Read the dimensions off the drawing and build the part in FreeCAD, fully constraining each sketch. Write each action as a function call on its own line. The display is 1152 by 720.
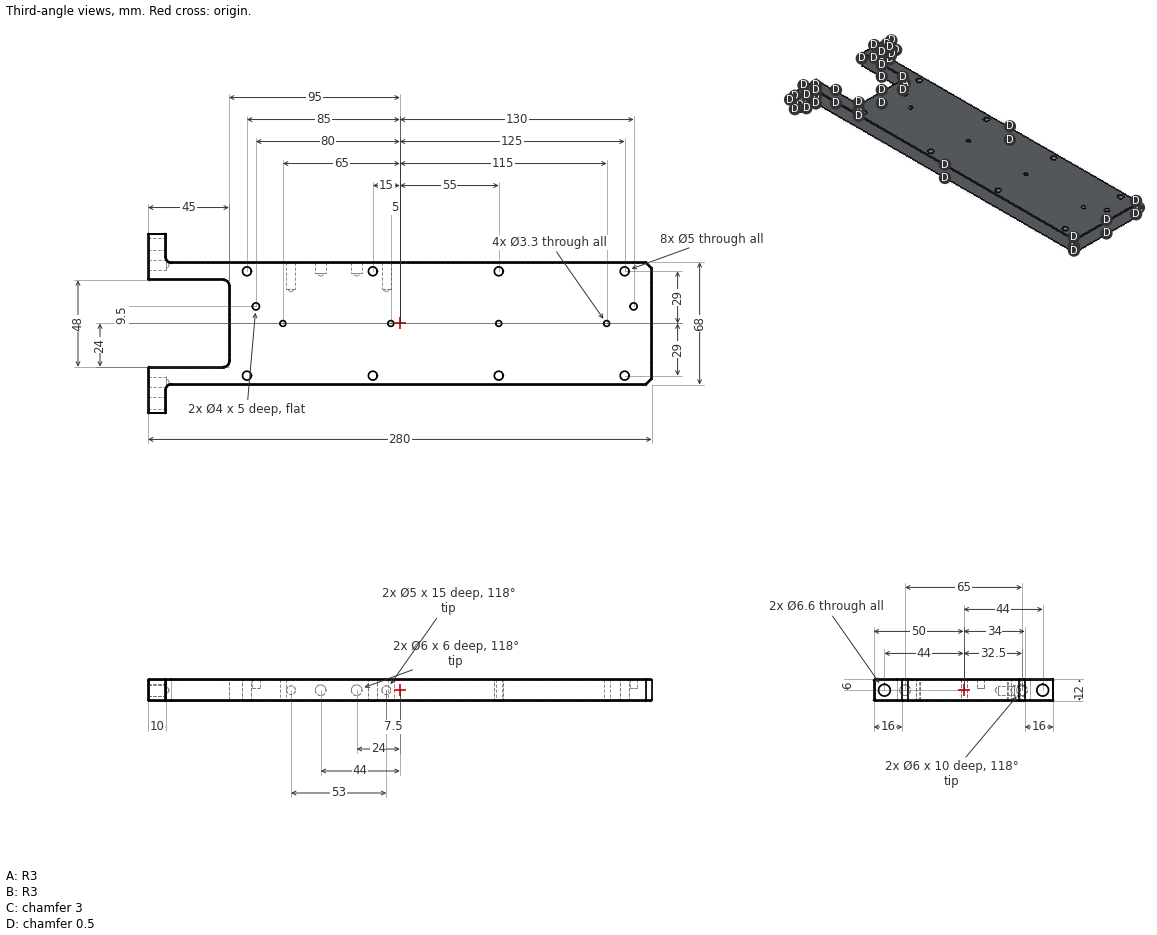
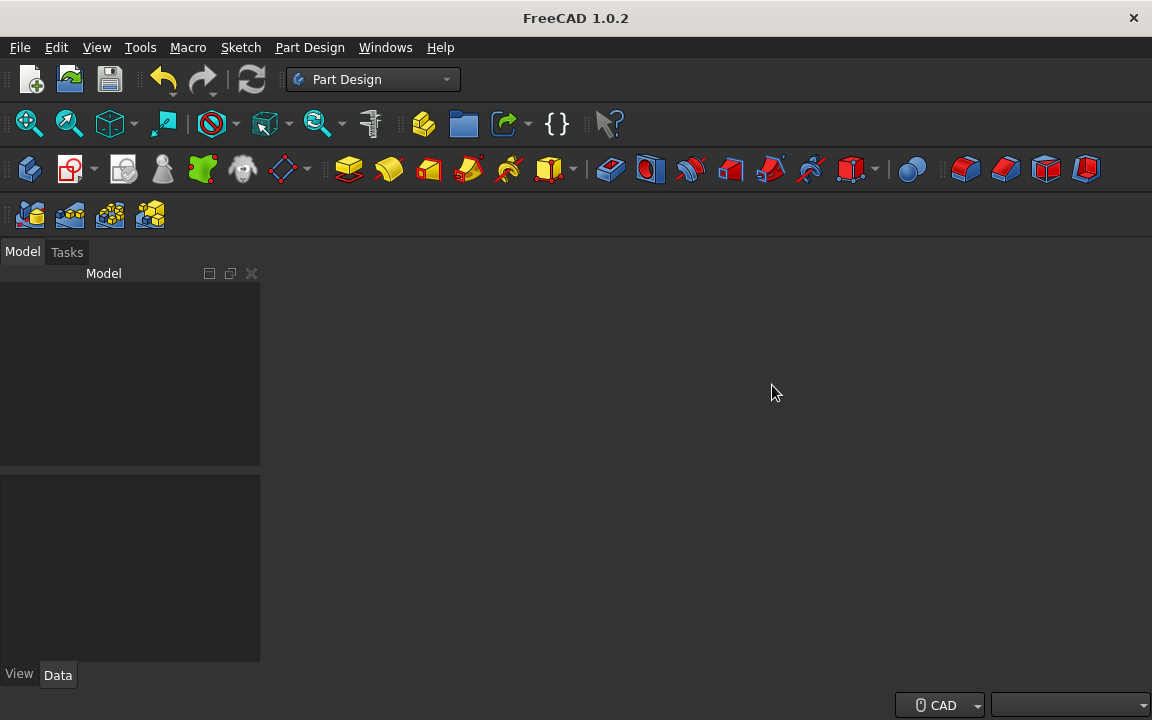
key(ctrl+n)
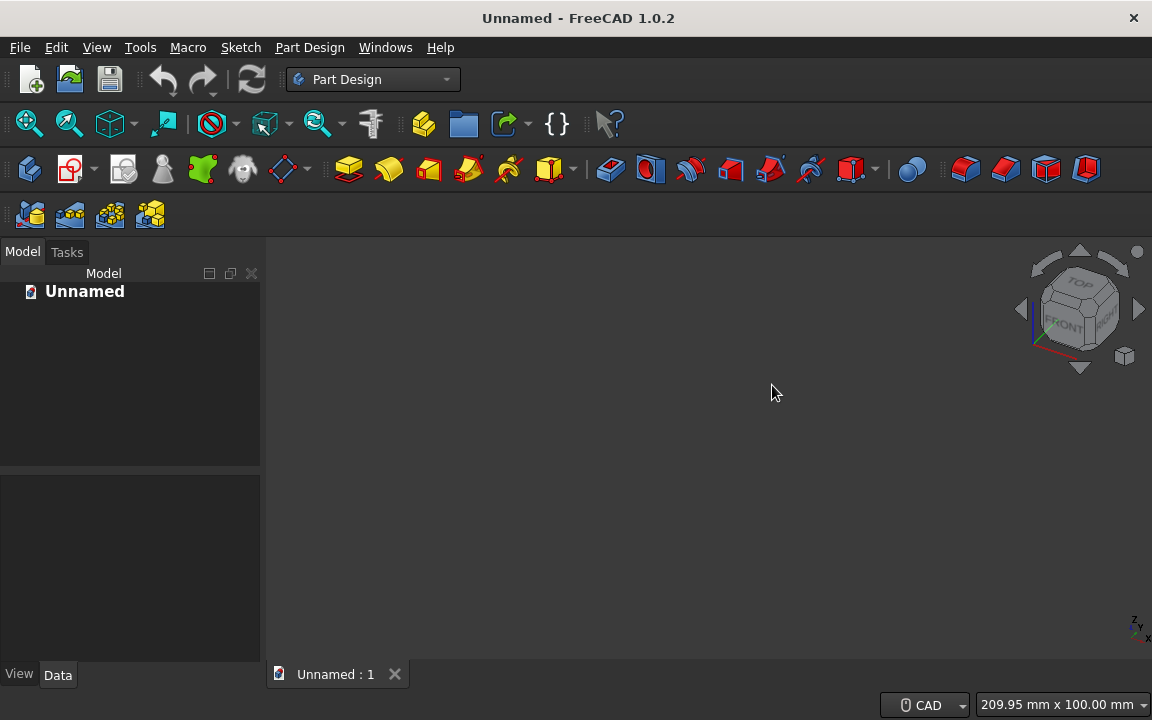
click(70, 170)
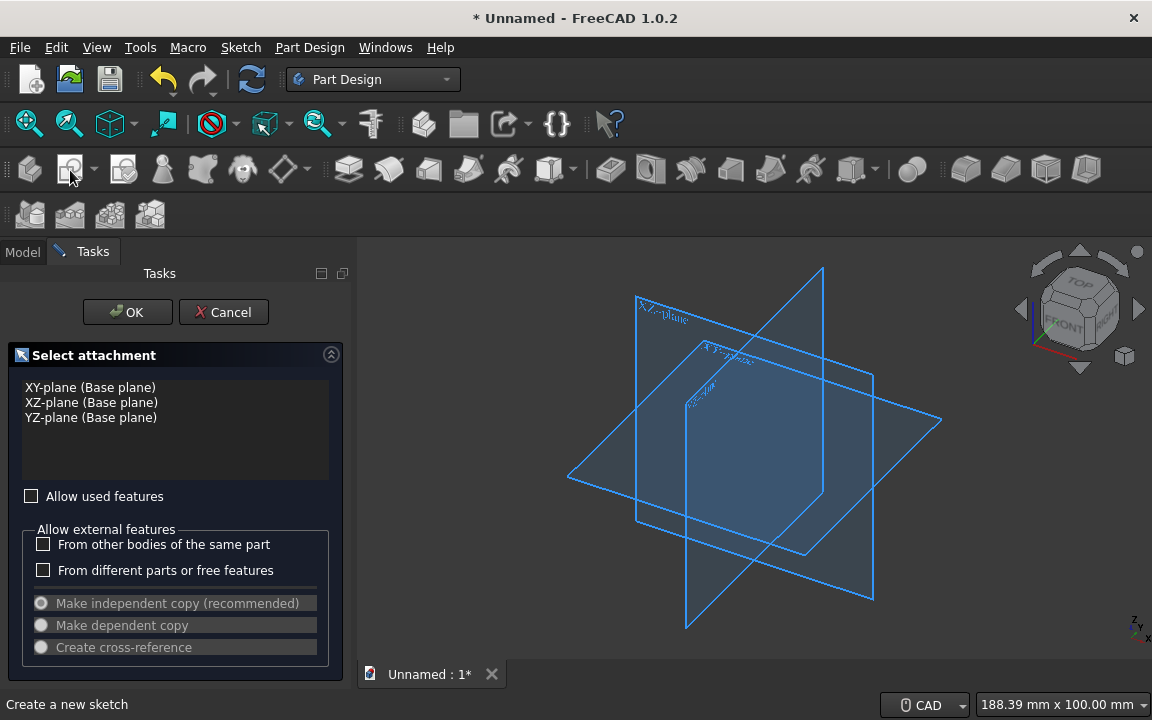
click(82, 388)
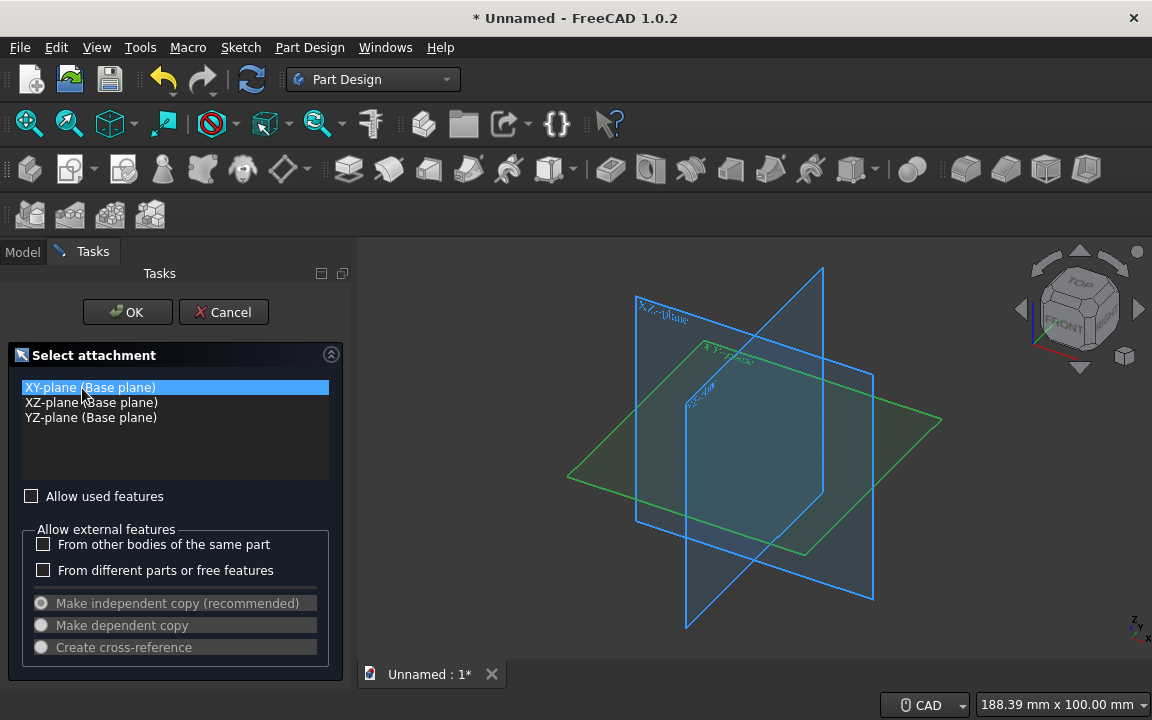
click(128, 312)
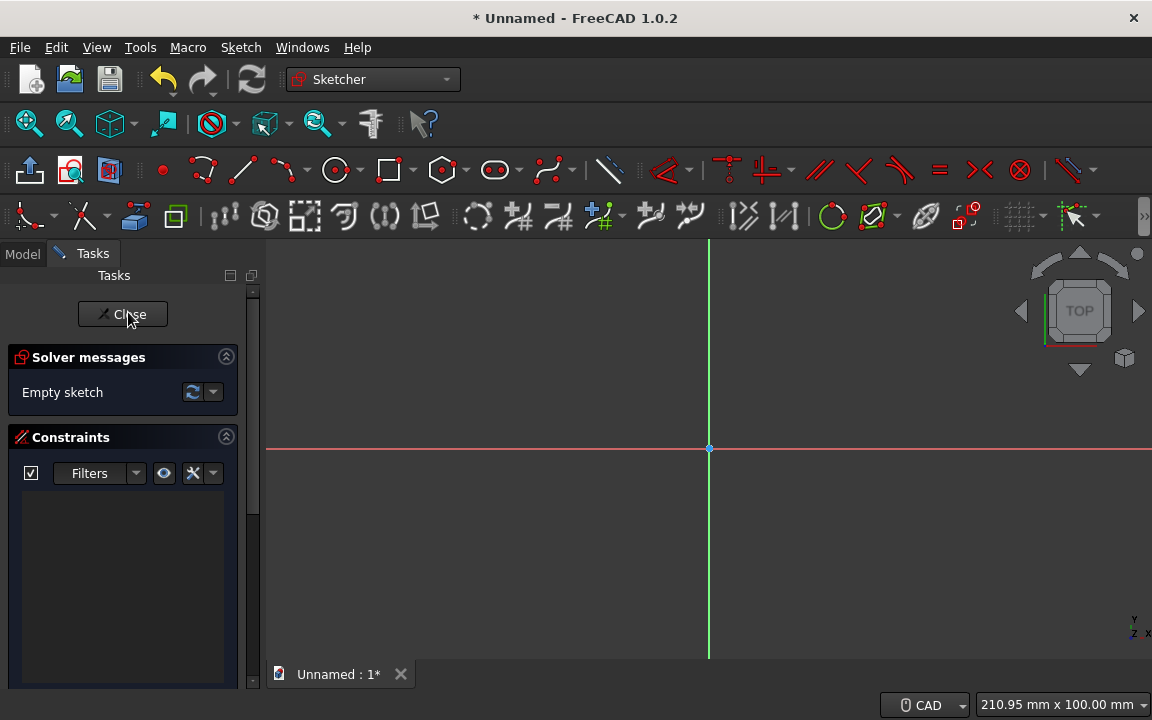
scroll(585, 449, down, 4)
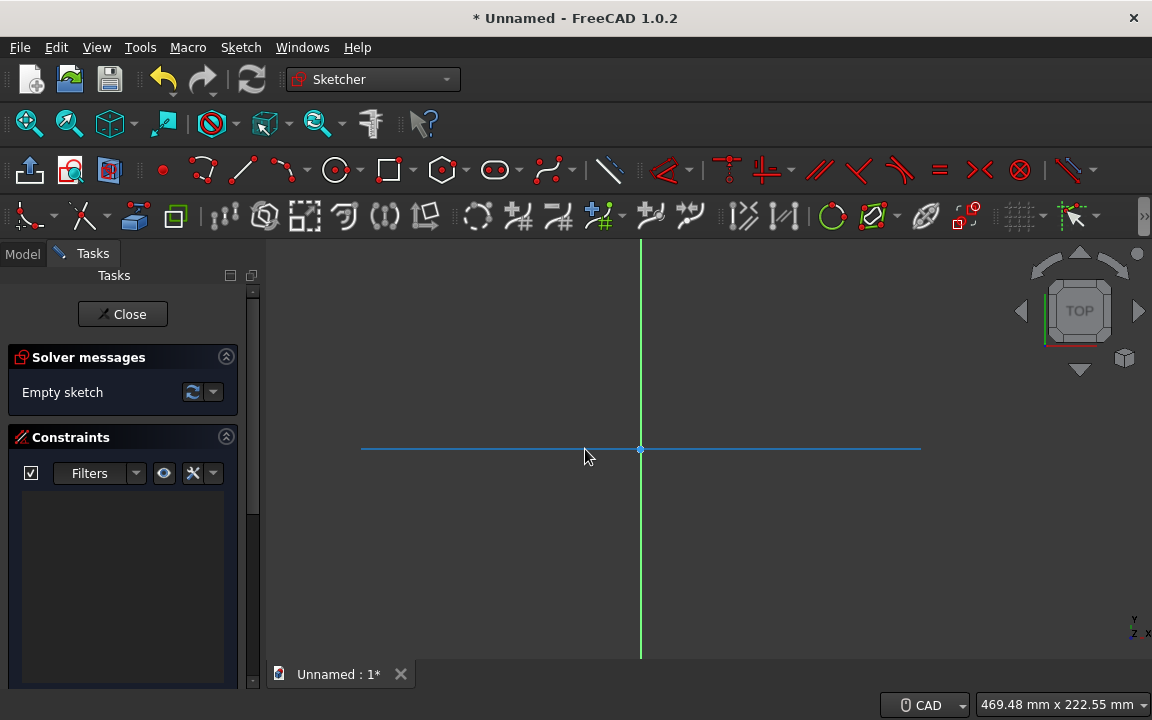
key(g)
key(v)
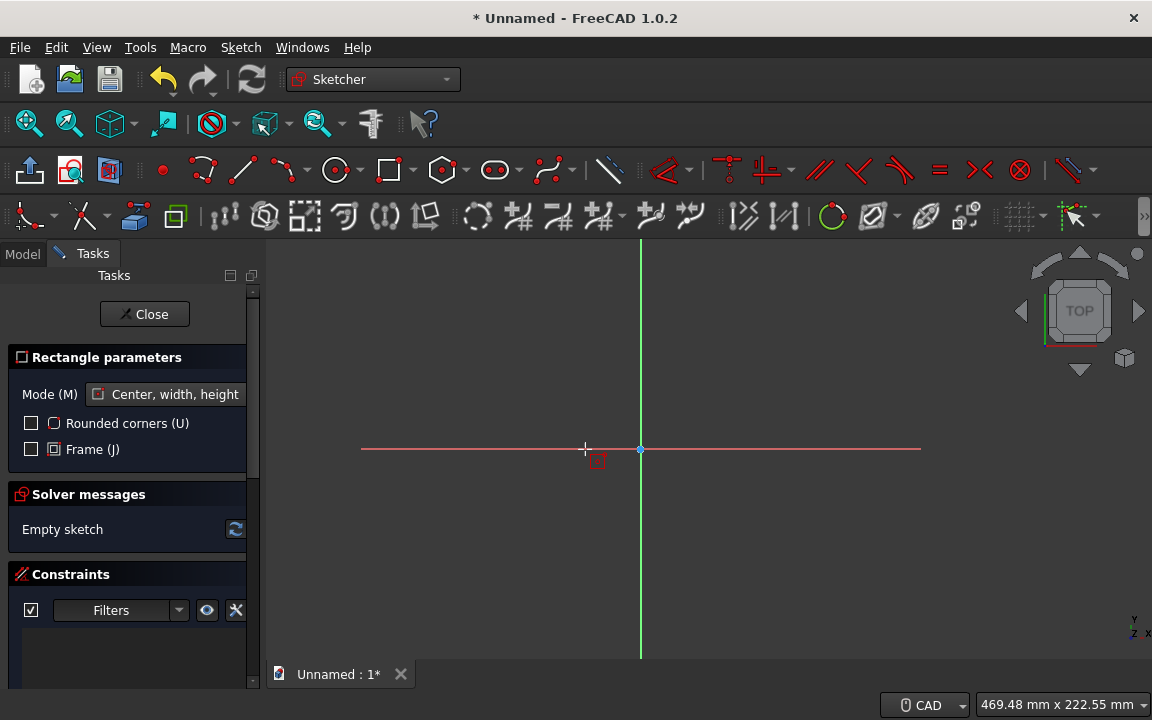
click(641, 449)
move(905, 385)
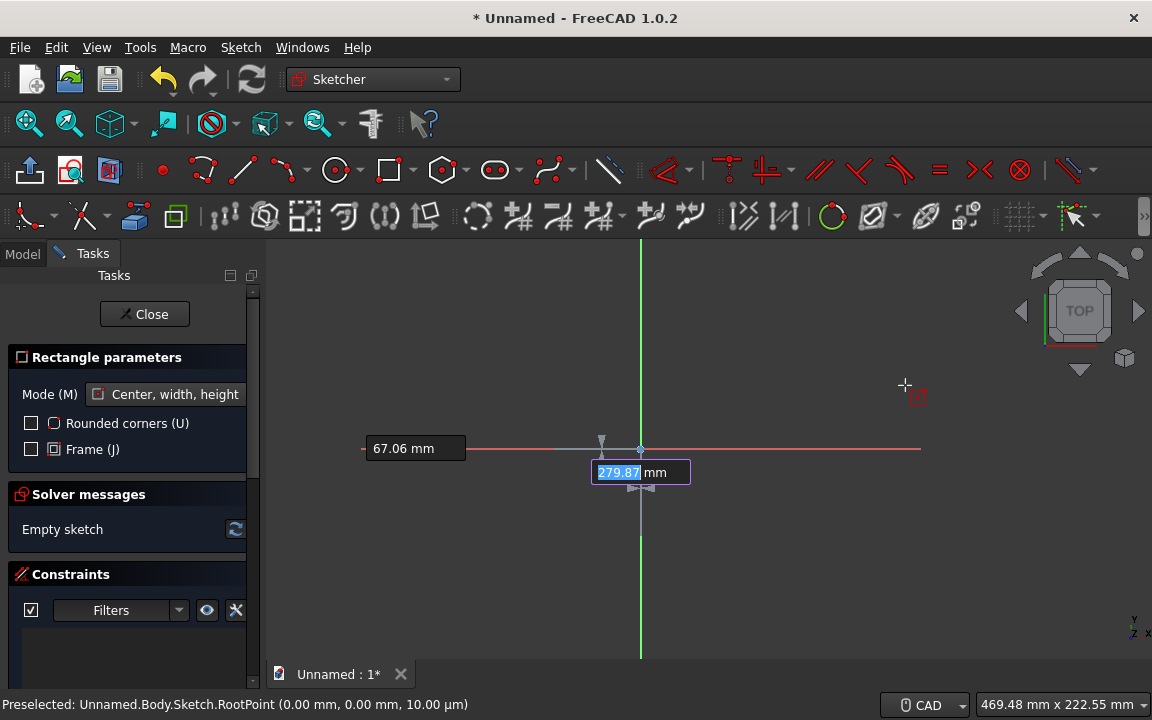
text(280)
key(Tab)
text(68)
key(Return)
key(Escape)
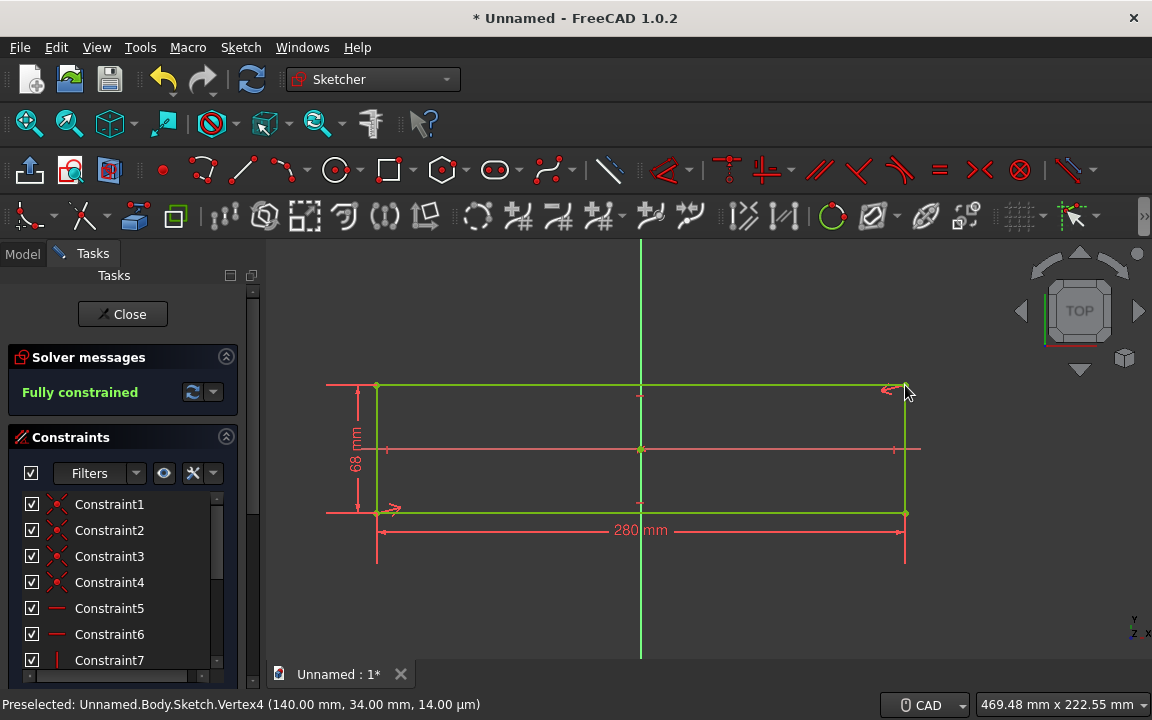
click(123, 314)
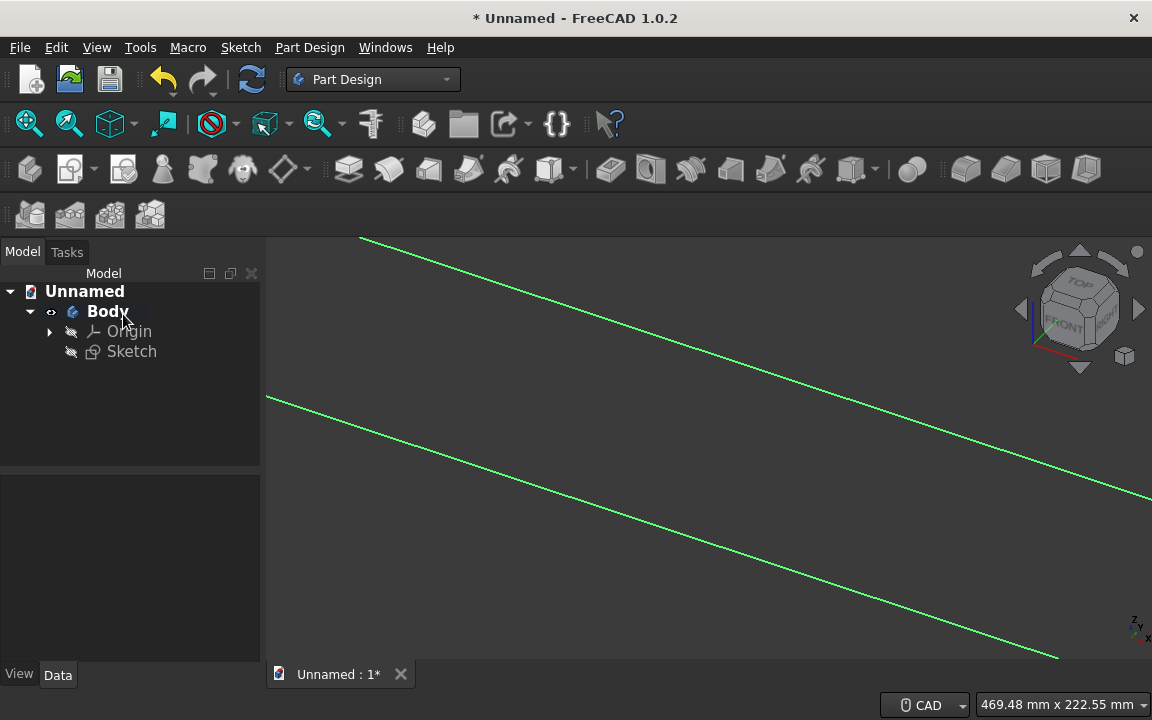
click(350, 170)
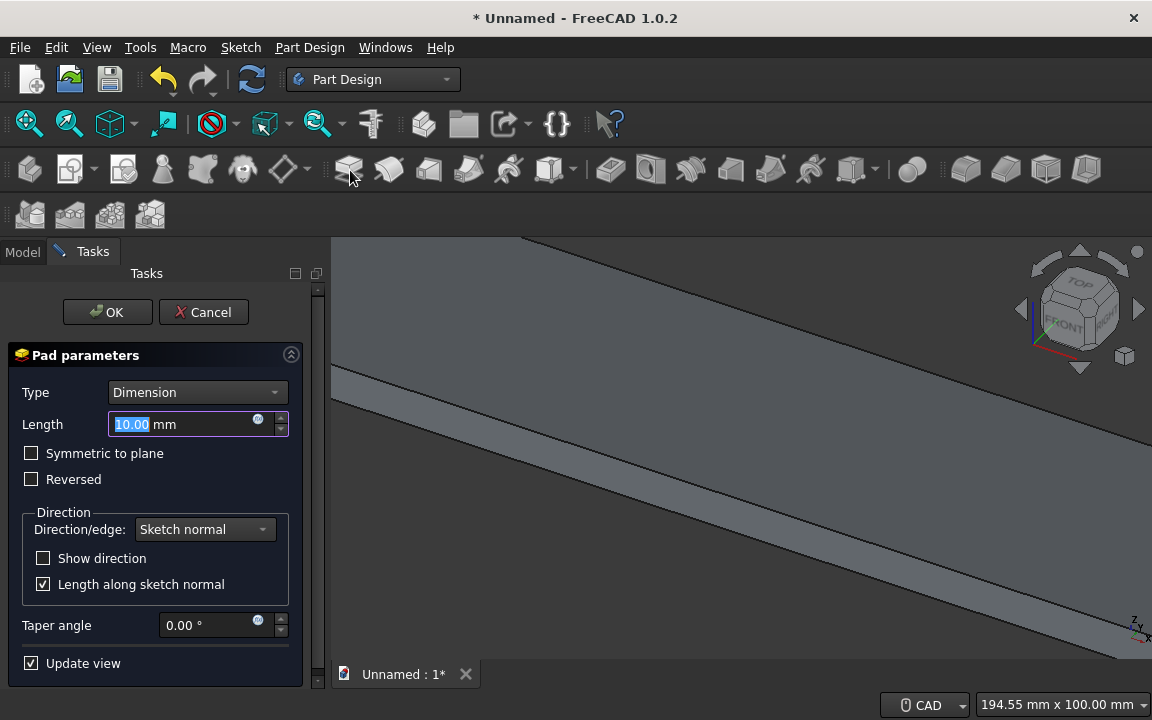
text(12)
key(Tab)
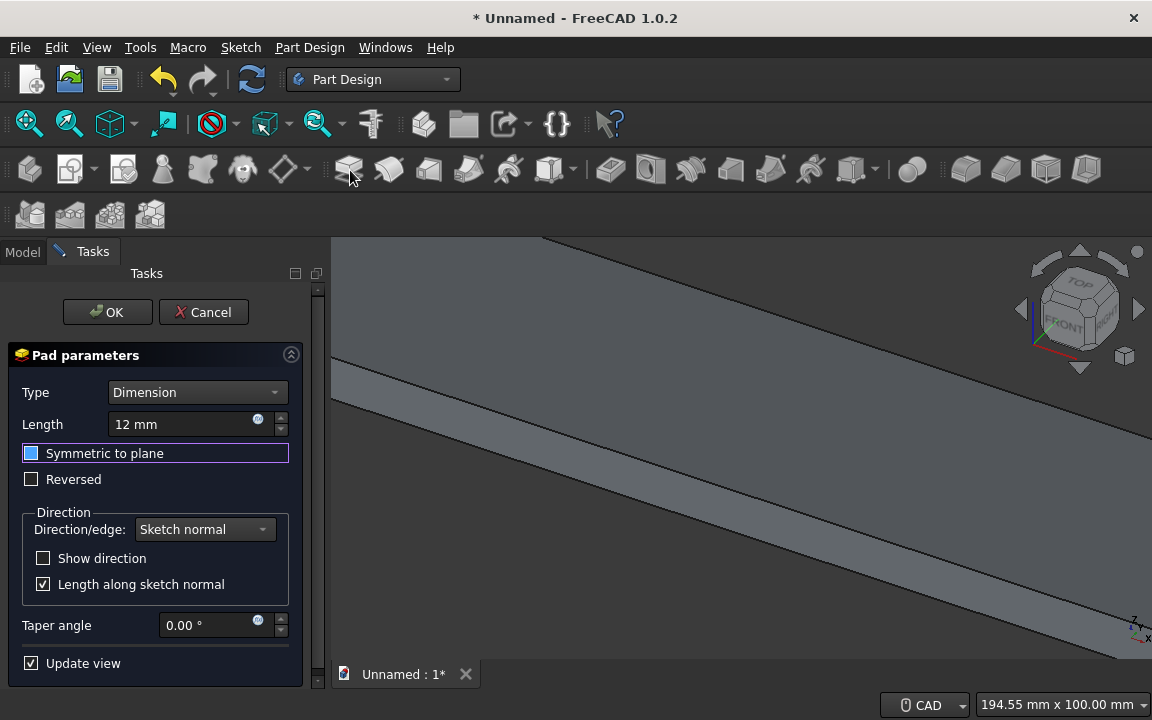
click(30, 453)